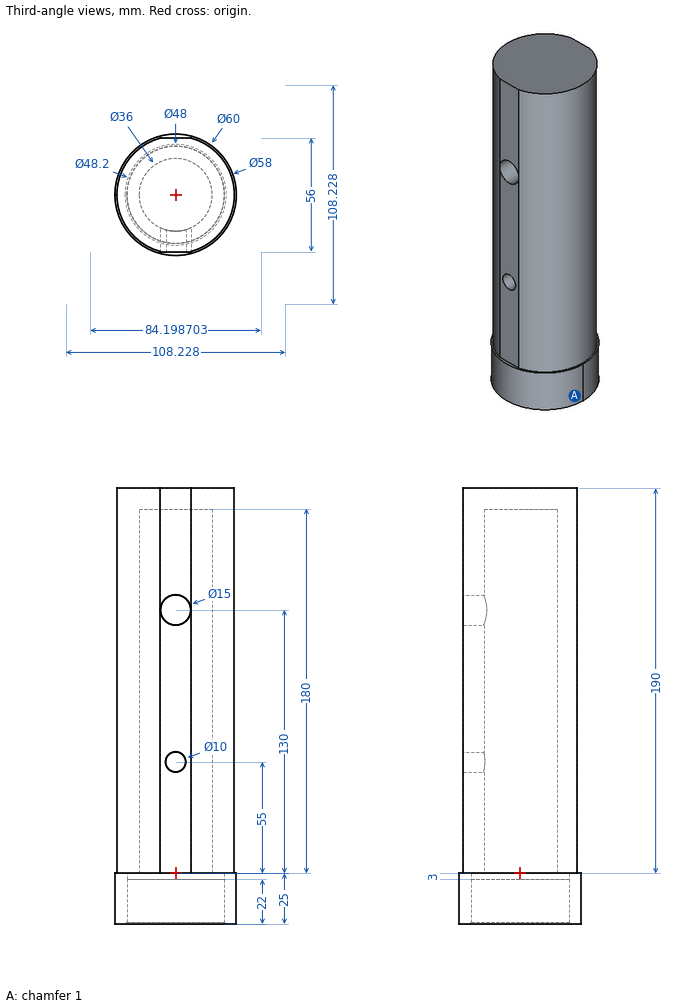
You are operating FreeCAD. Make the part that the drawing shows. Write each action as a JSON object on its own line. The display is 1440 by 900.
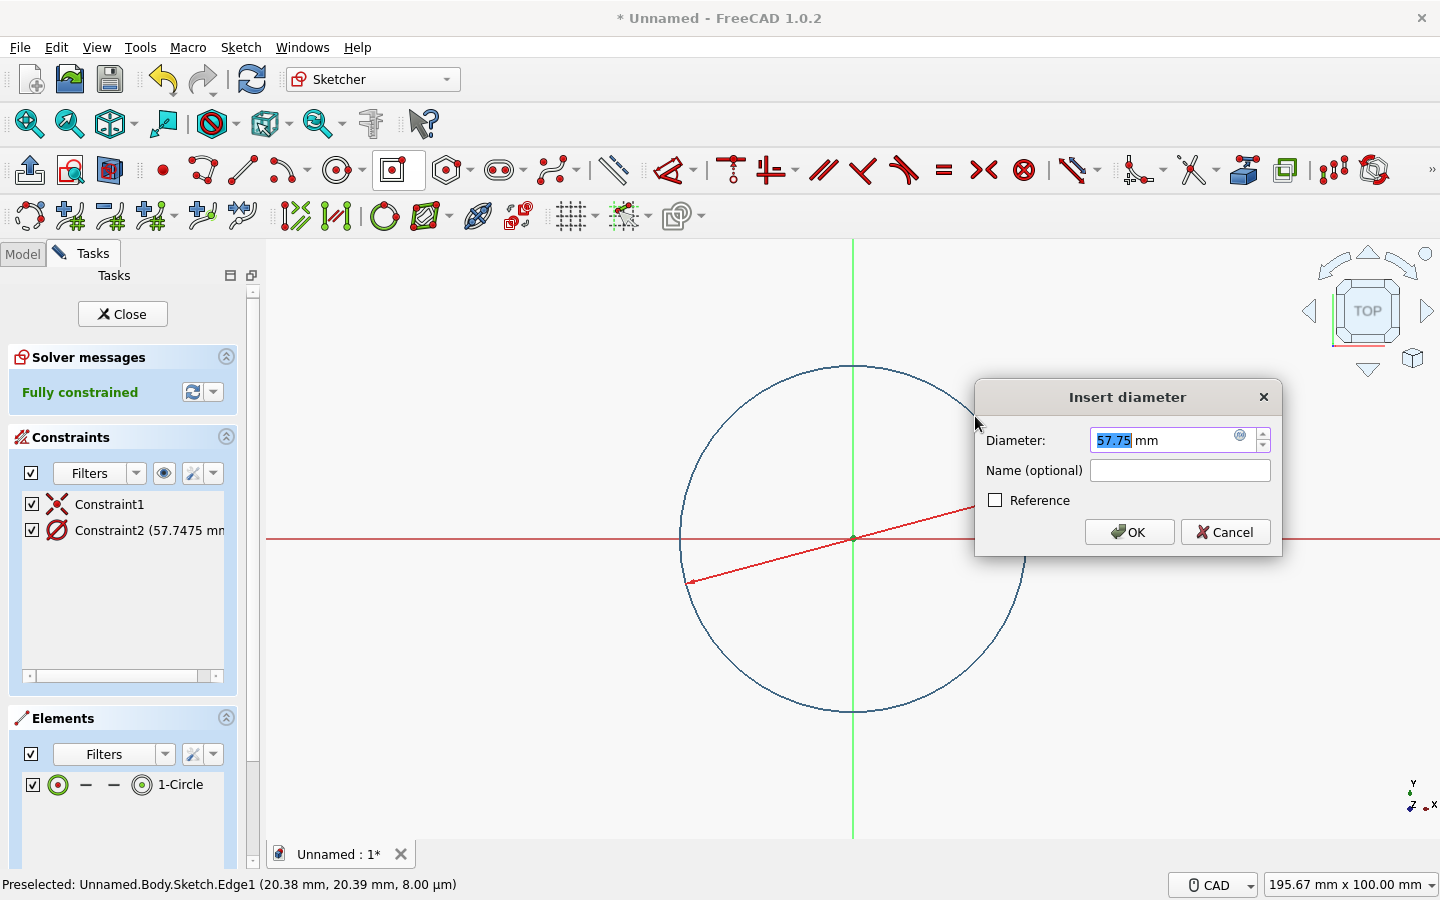
{"action": "type", "text": "58"}
{"action": "key", "text": "Return"}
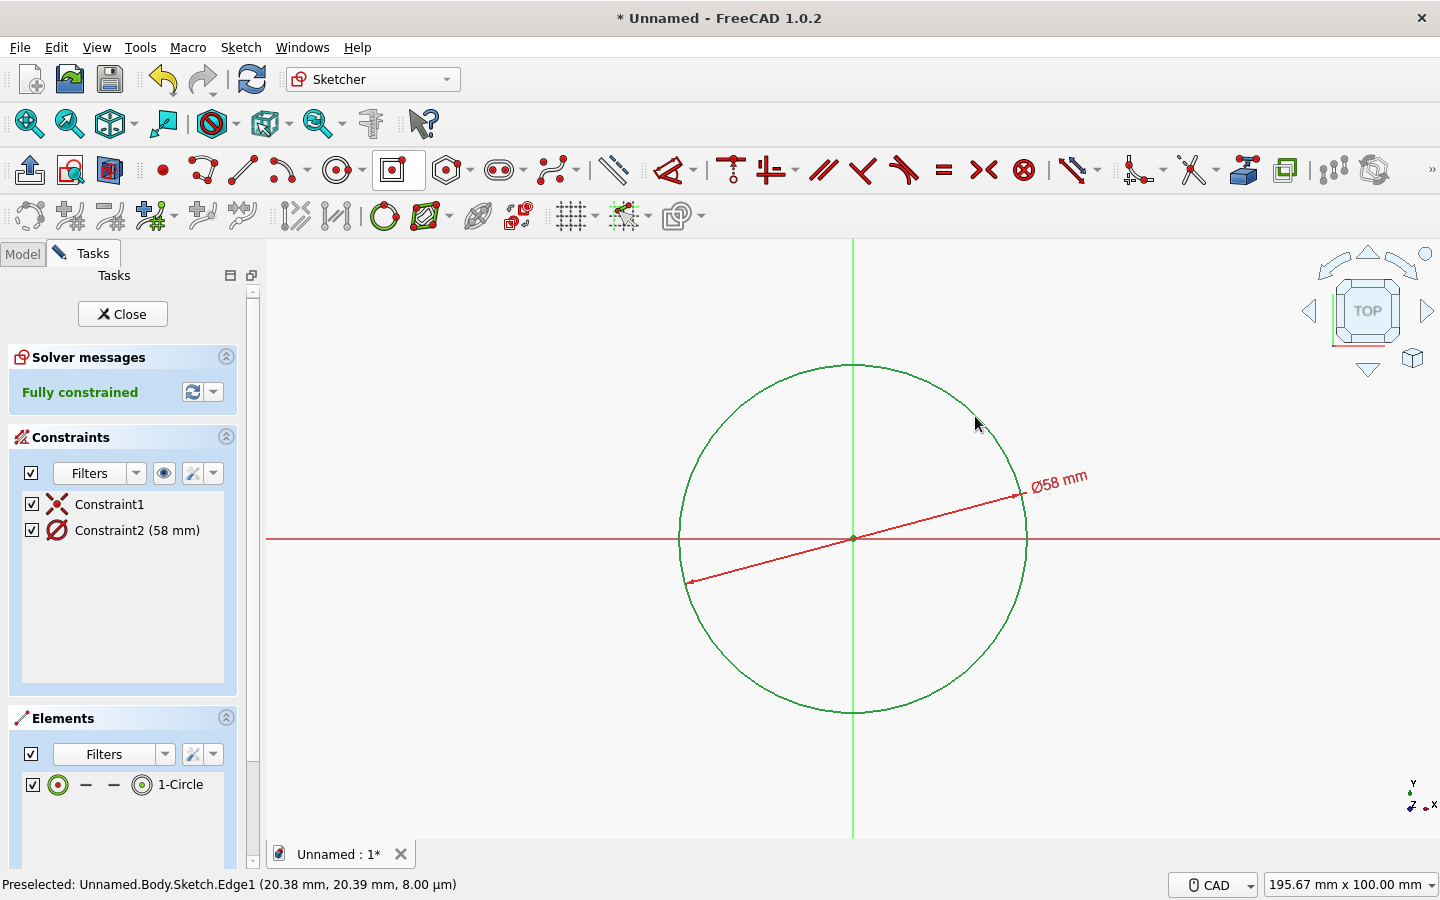
{"action": "left_click", "coordinate": [123, 314]}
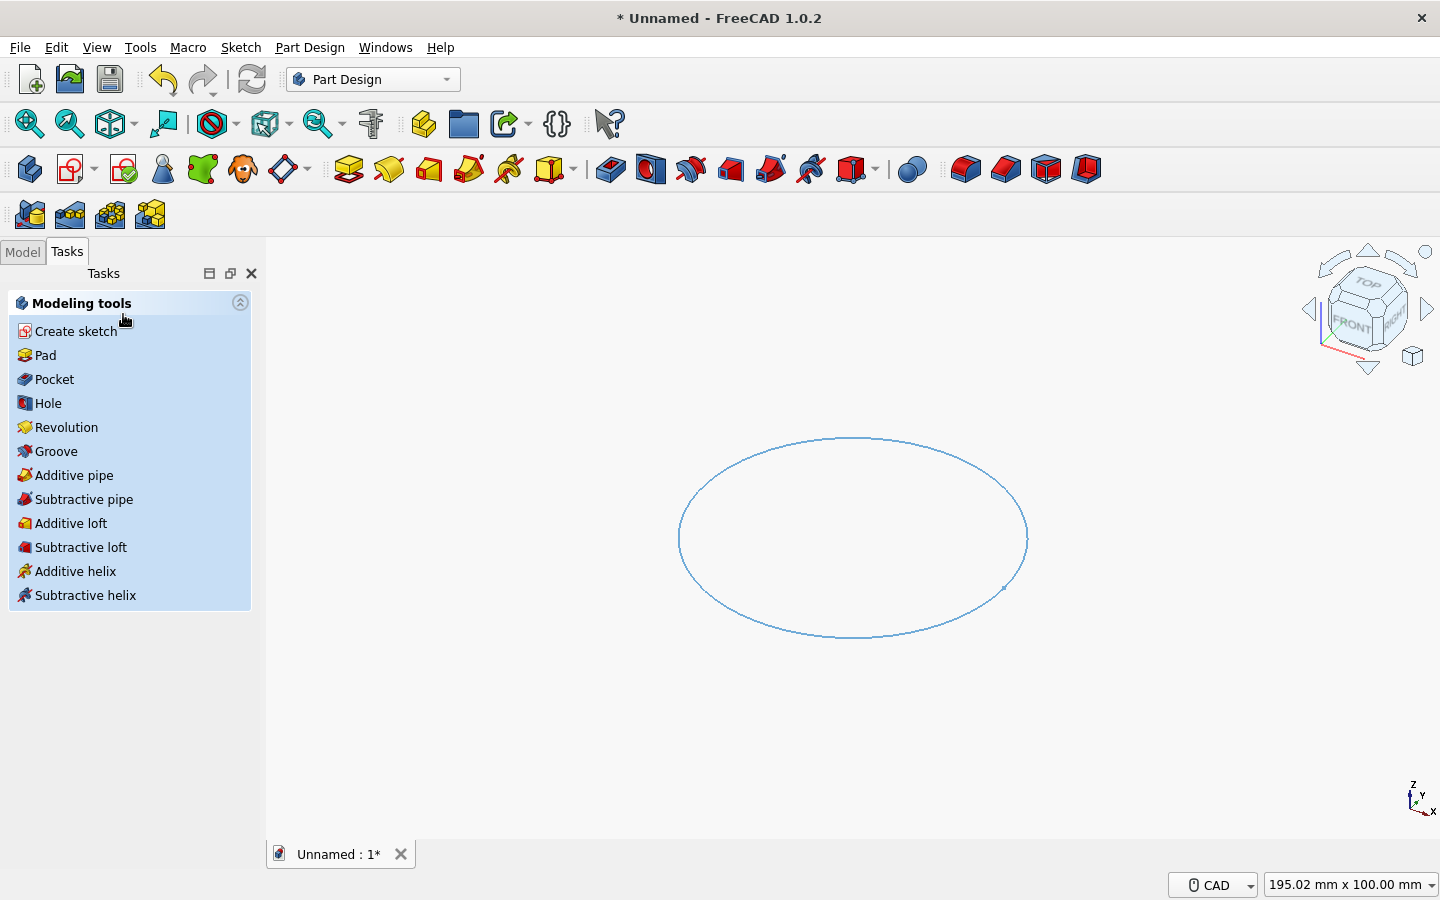
{"action": "left_click", "coordinate": [350, 170]}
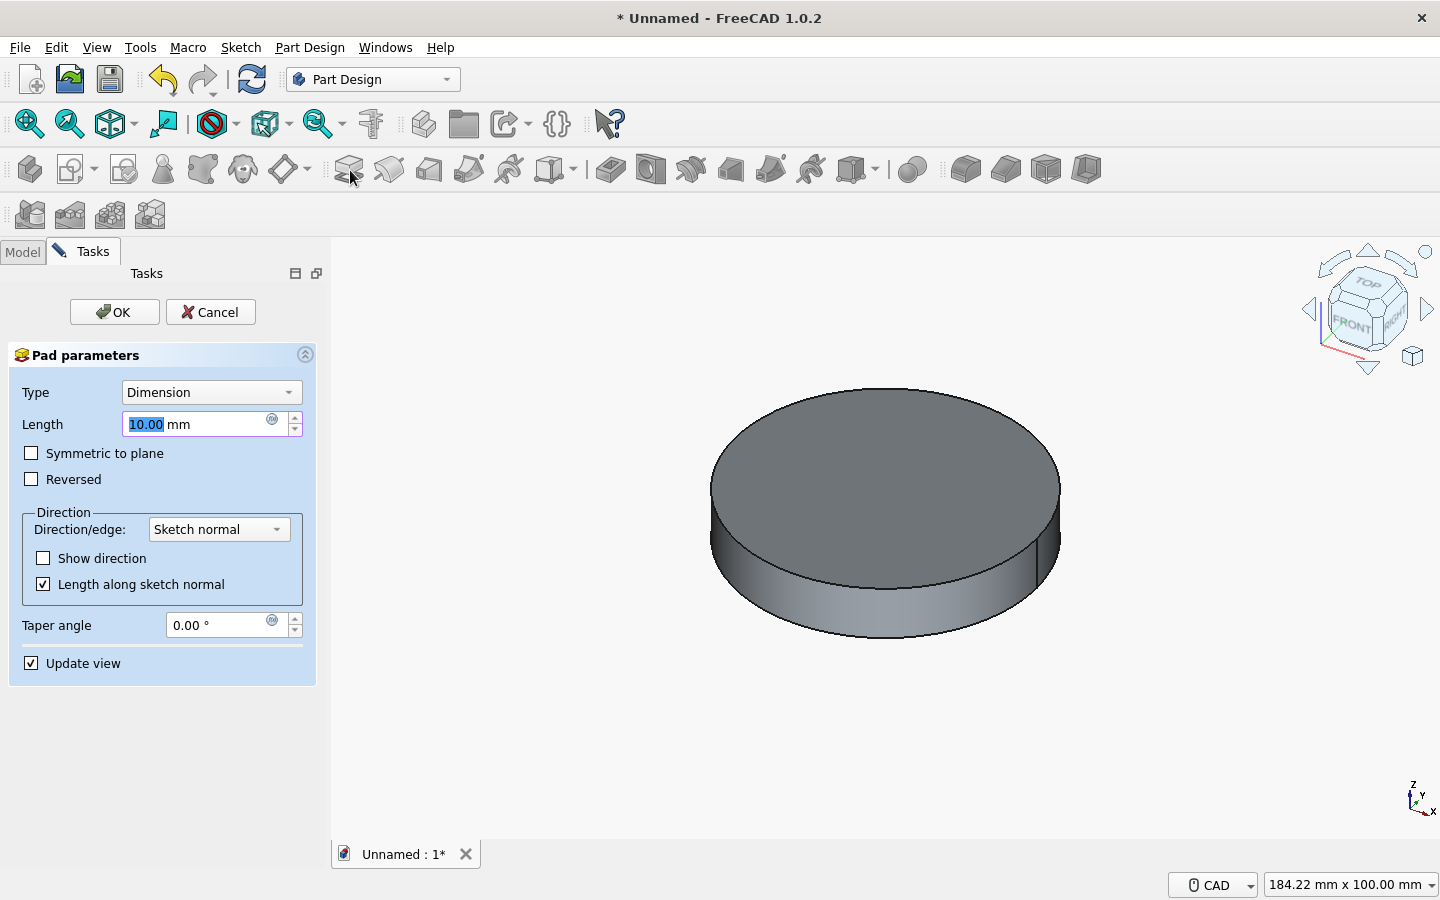
{"action": "type", "text": "190"}
{"action": "key", "text": "Tab"}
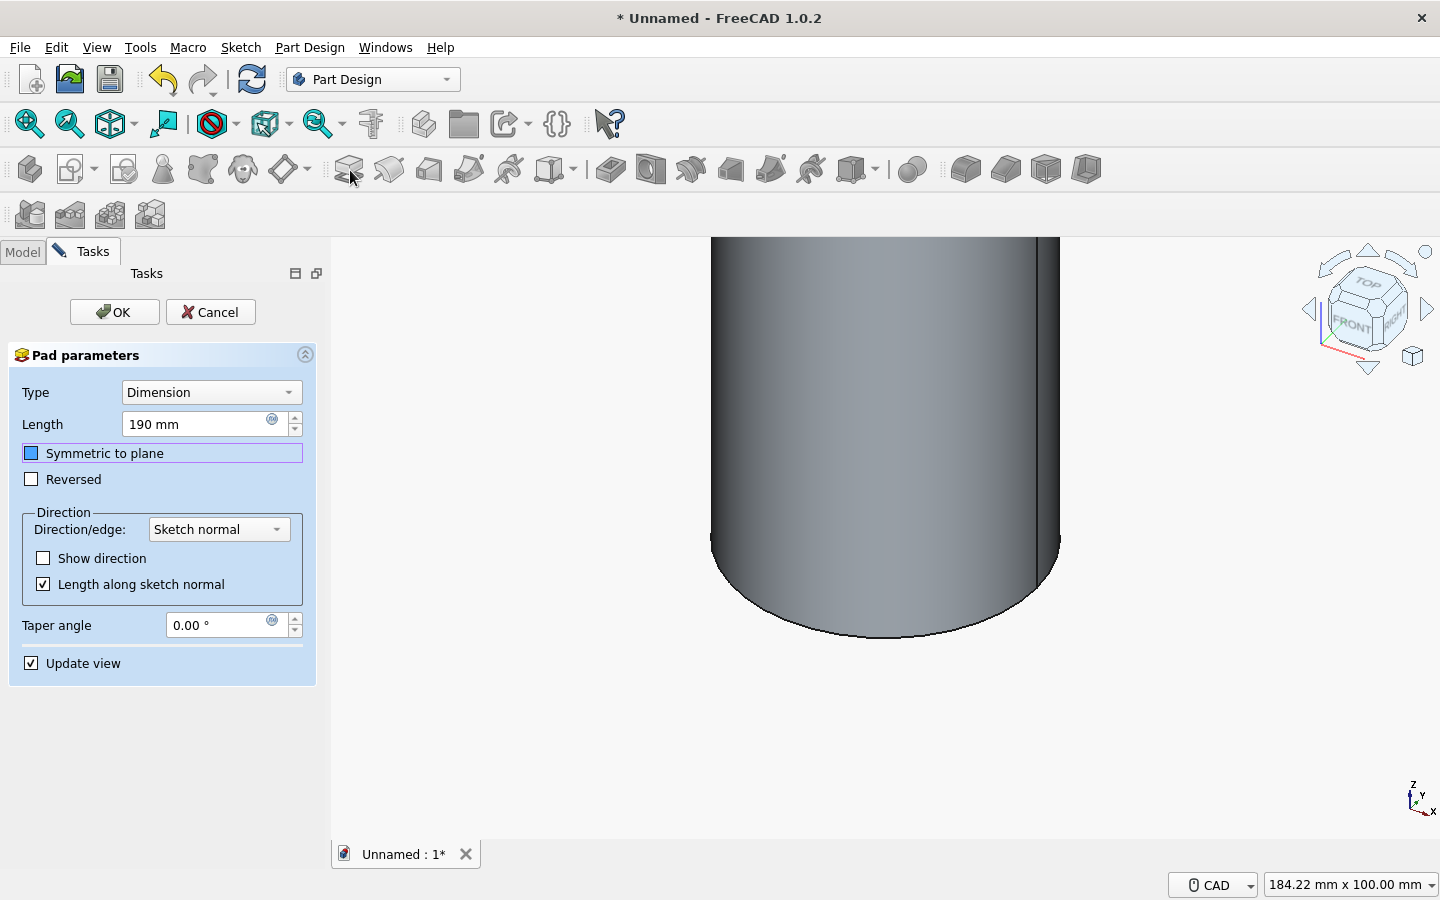
{"action": "left_click", "coordinate": [115, 312]}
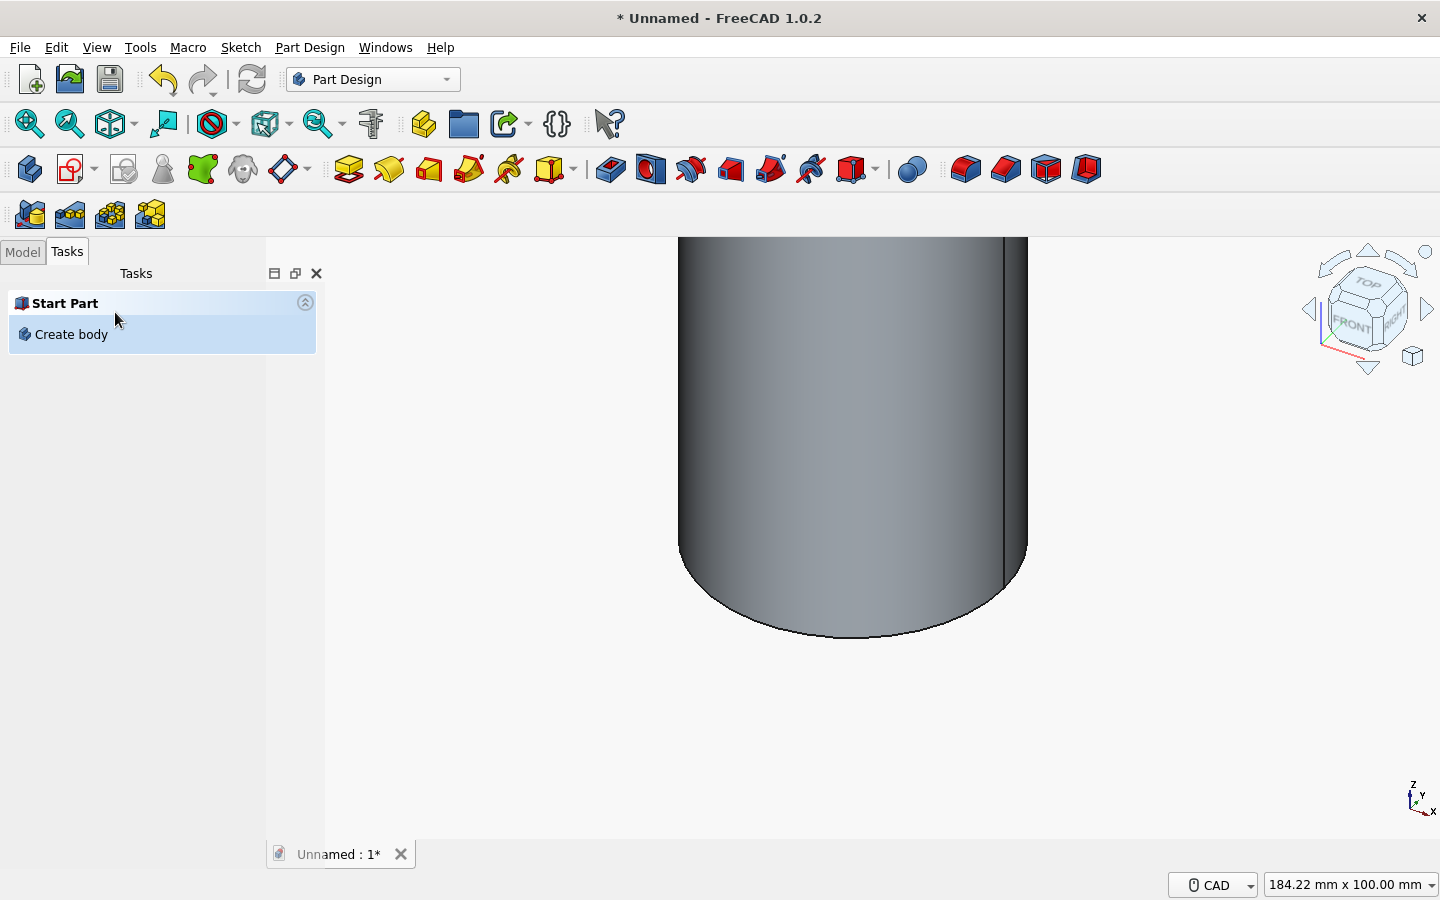
{"action": "left_click", "coordinate": [30, 124]}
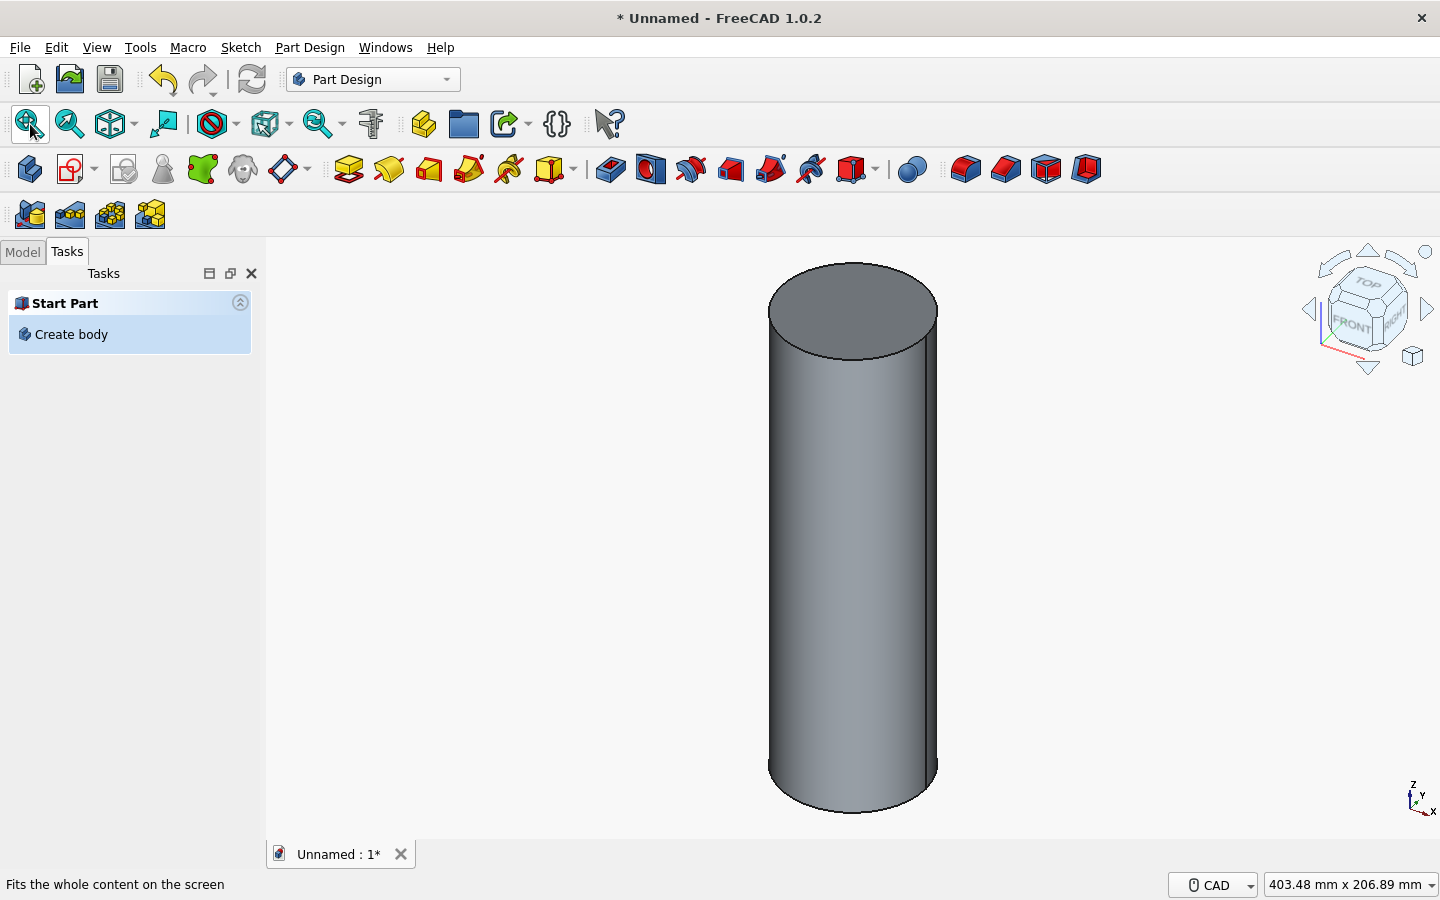
{"action": "left_click", "coordinate": [70, 170]}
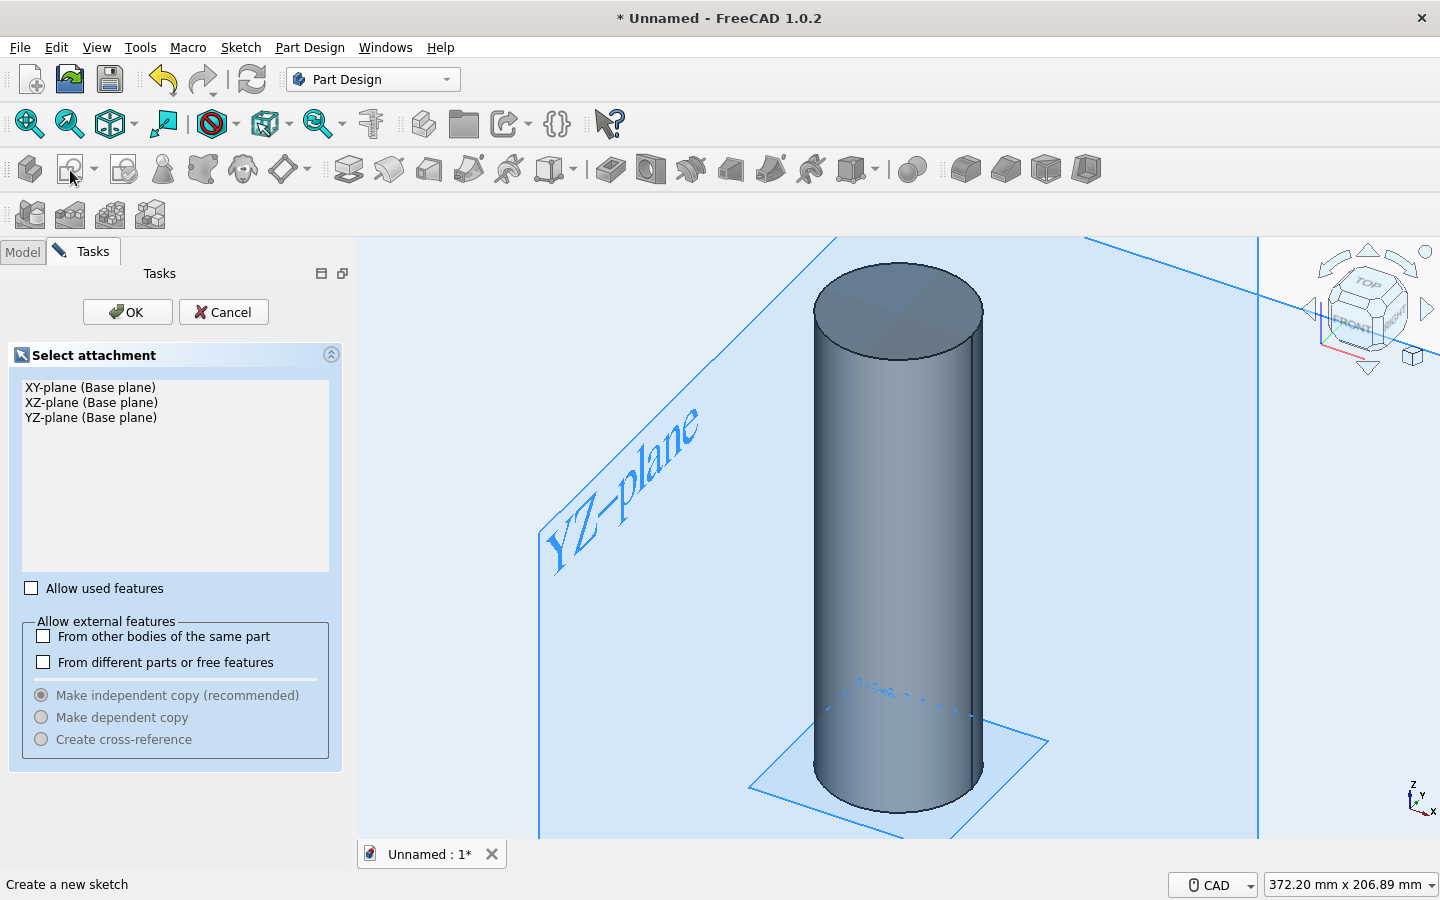
{"action": "left_click", "coordinate": [82, 388]}